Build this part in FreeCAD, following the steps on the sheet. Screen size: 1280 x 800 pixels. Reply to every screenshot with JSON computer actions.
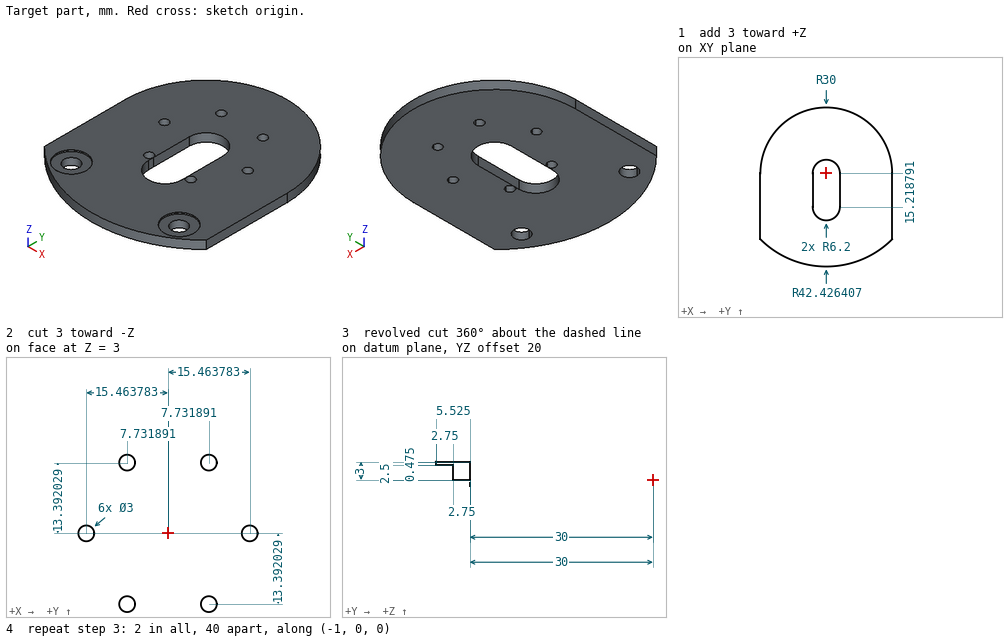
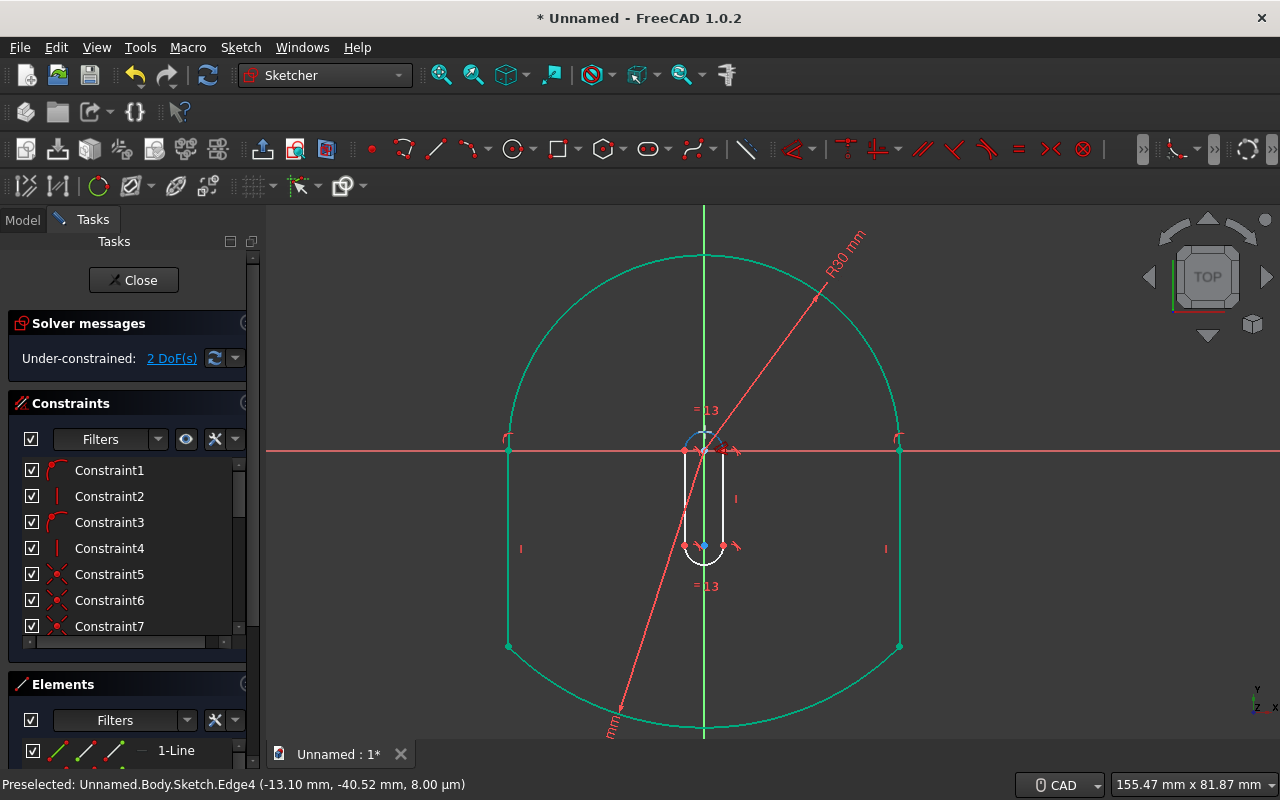
{"action": "left_click", "coordinate": [704, 432]}
{"action": "left_click", "coordinate": [728, 406]}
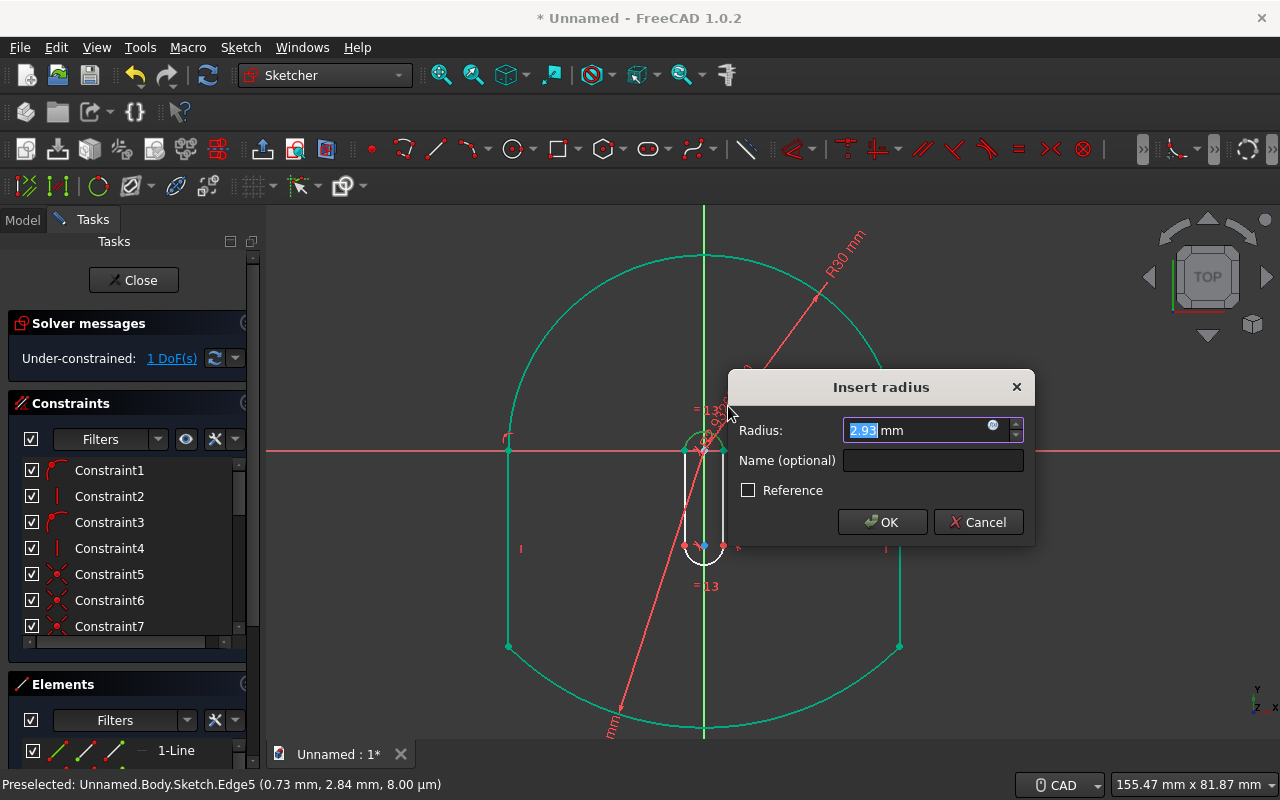
{"action": "type", "text": "6.2"}
{"action": "key", "text": "Return"}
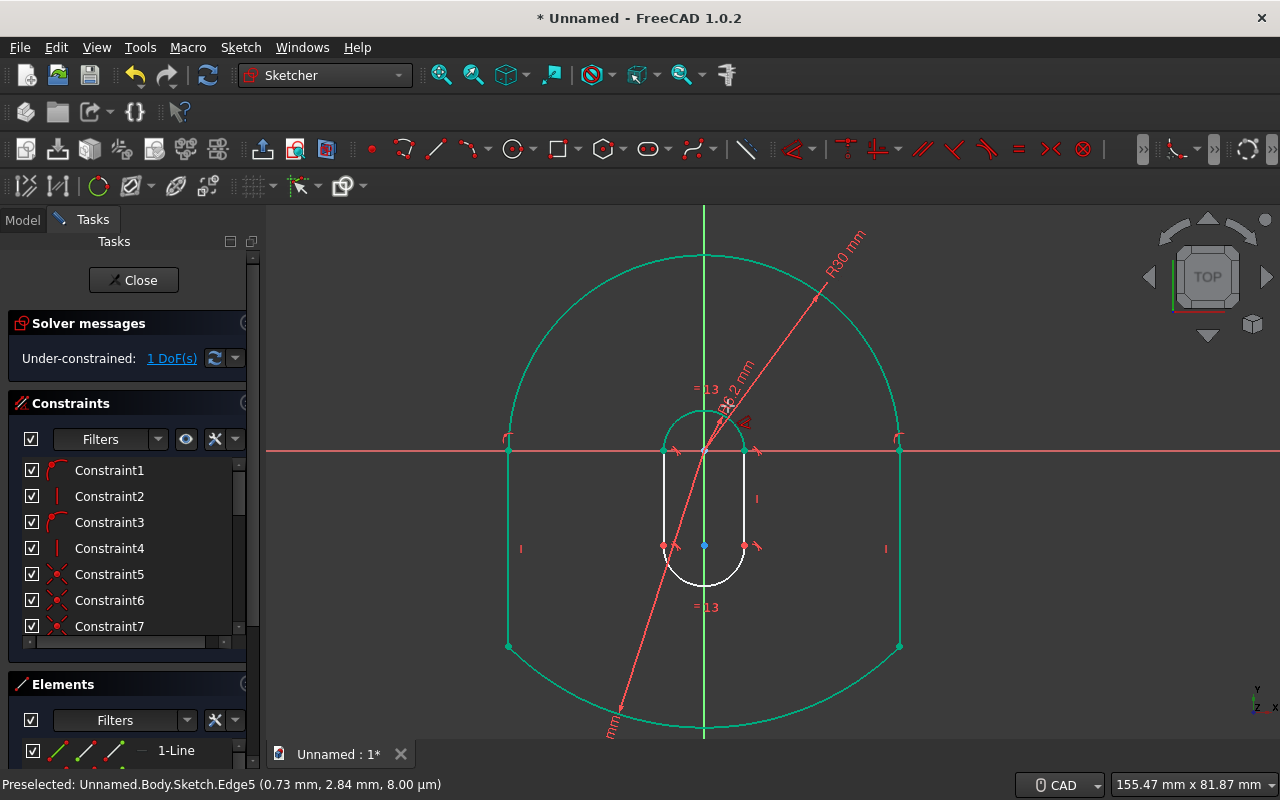
{"action": "left_click", "coordinate": [744, 479]}
{"action": "left_click", "coordinate": [778, 498]}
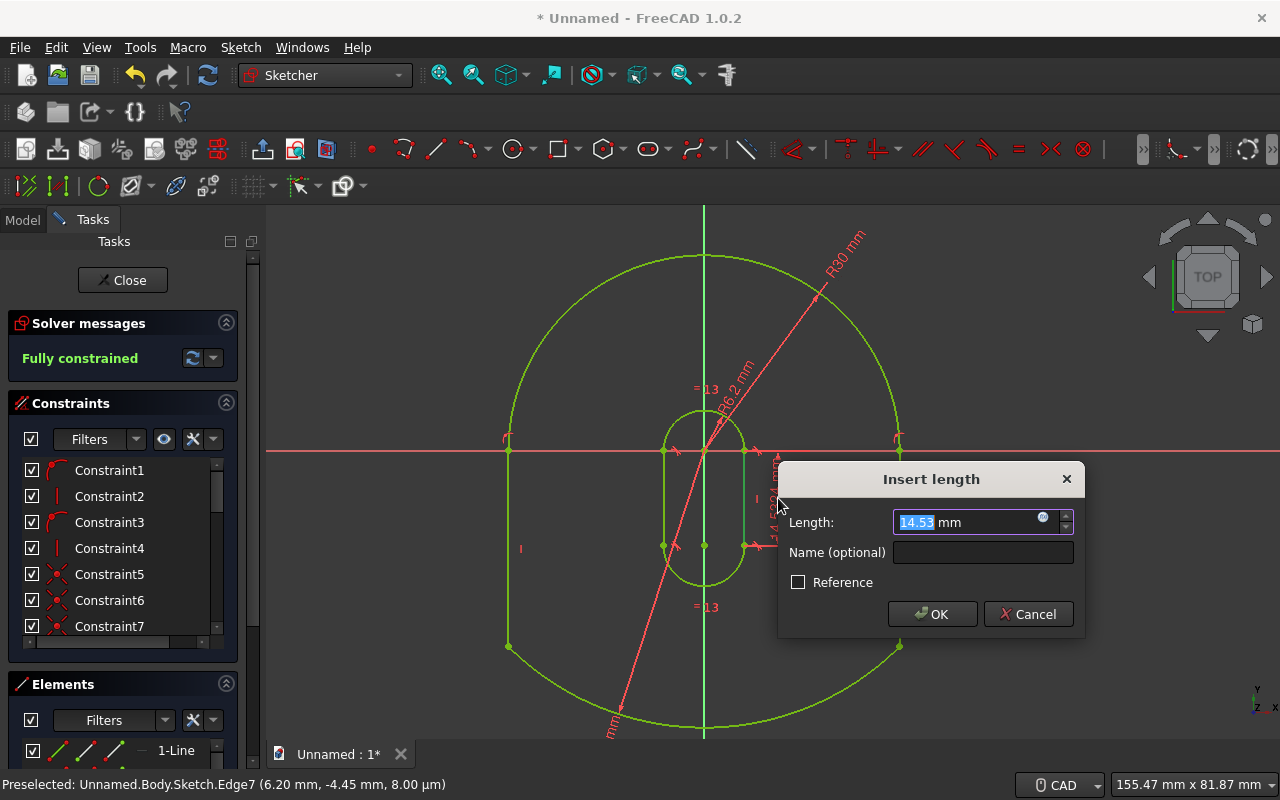
{"action": "type", "text": "15.218791"}
{"action": "key", "text": "Return"}
{"action": "key", "text": "Escape"}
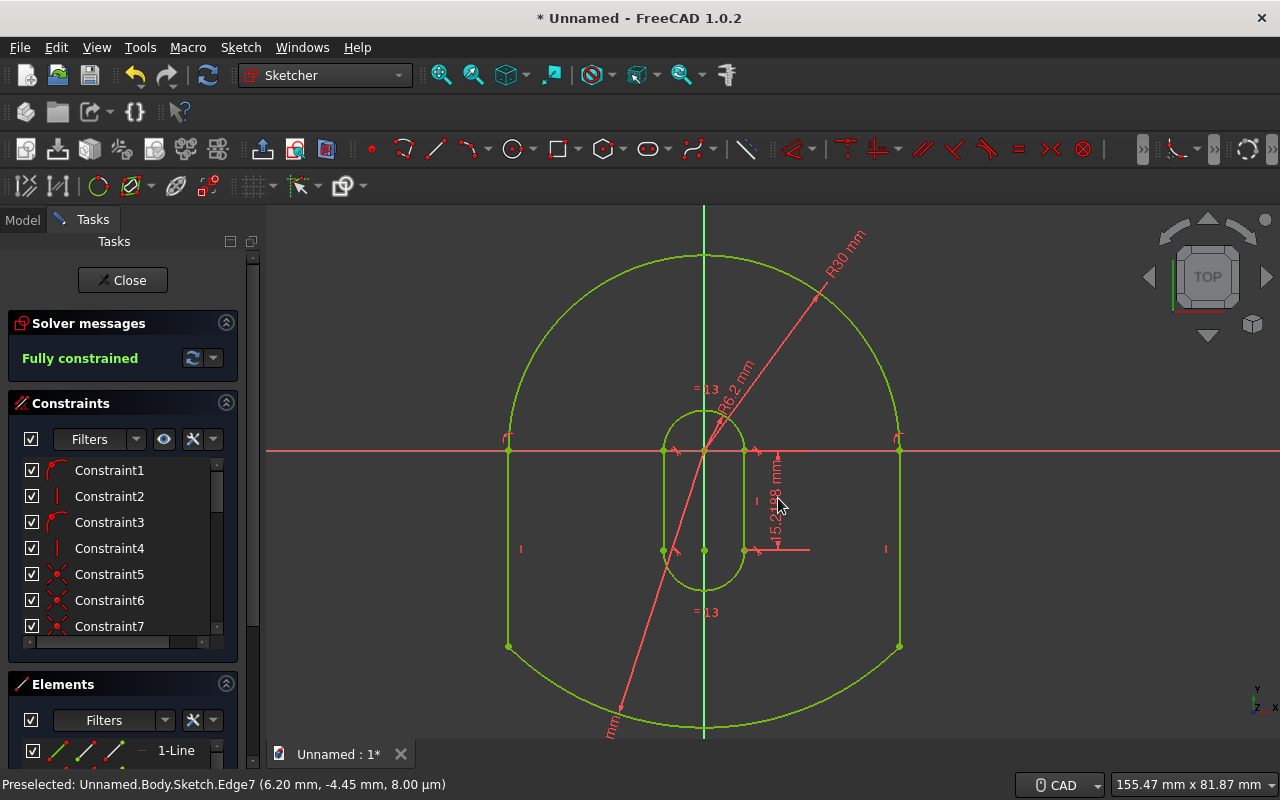
{"action": "left_click", "coordinate": [123, 280]}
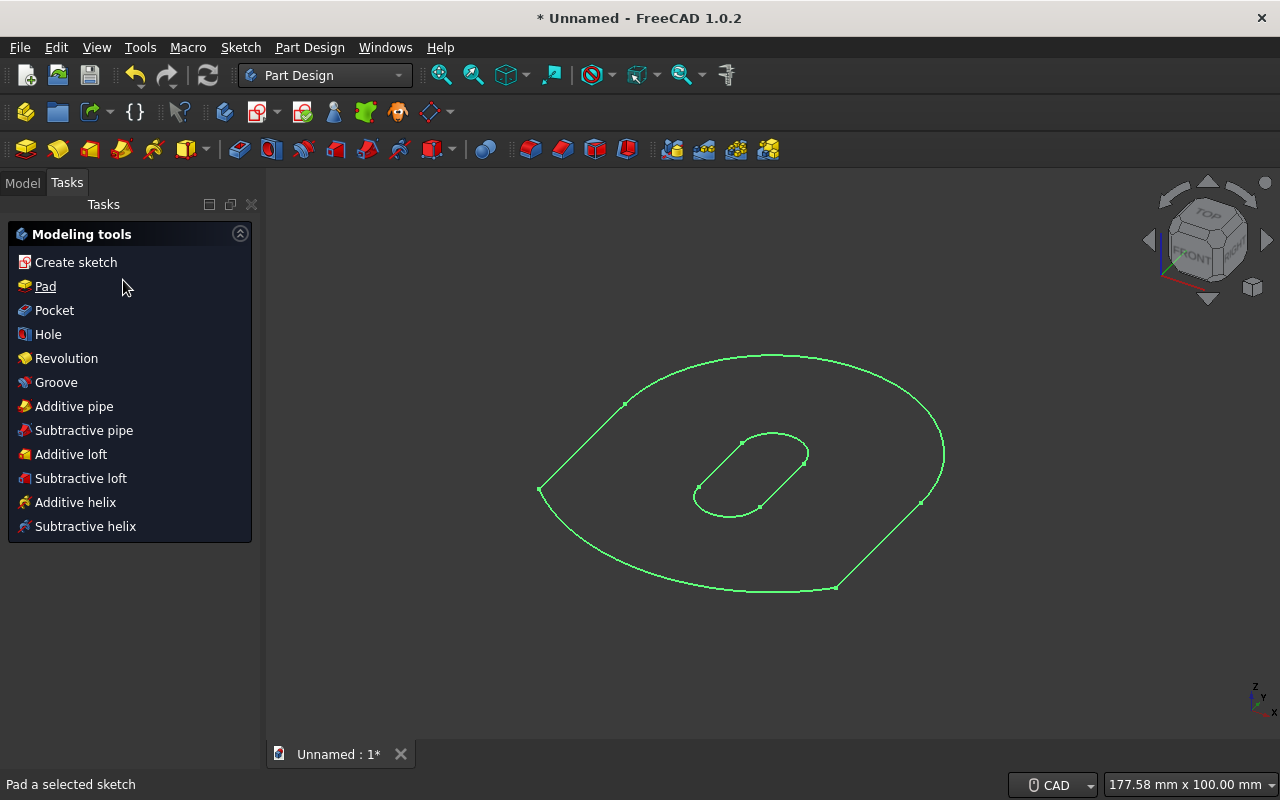
{"action": "left_click", "coordinate": [26, 150]}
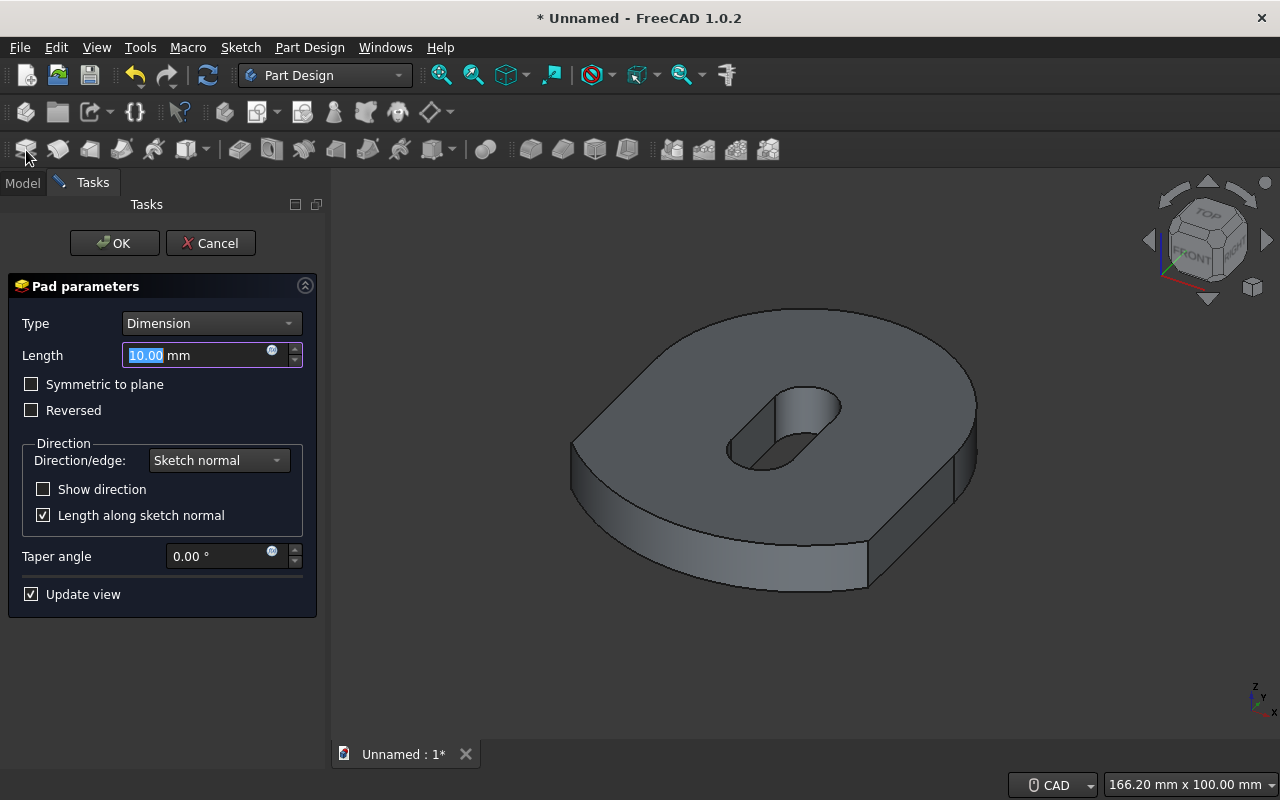
{"action": "type", "text": "3"}
{"action": "key", "text": "Tab"}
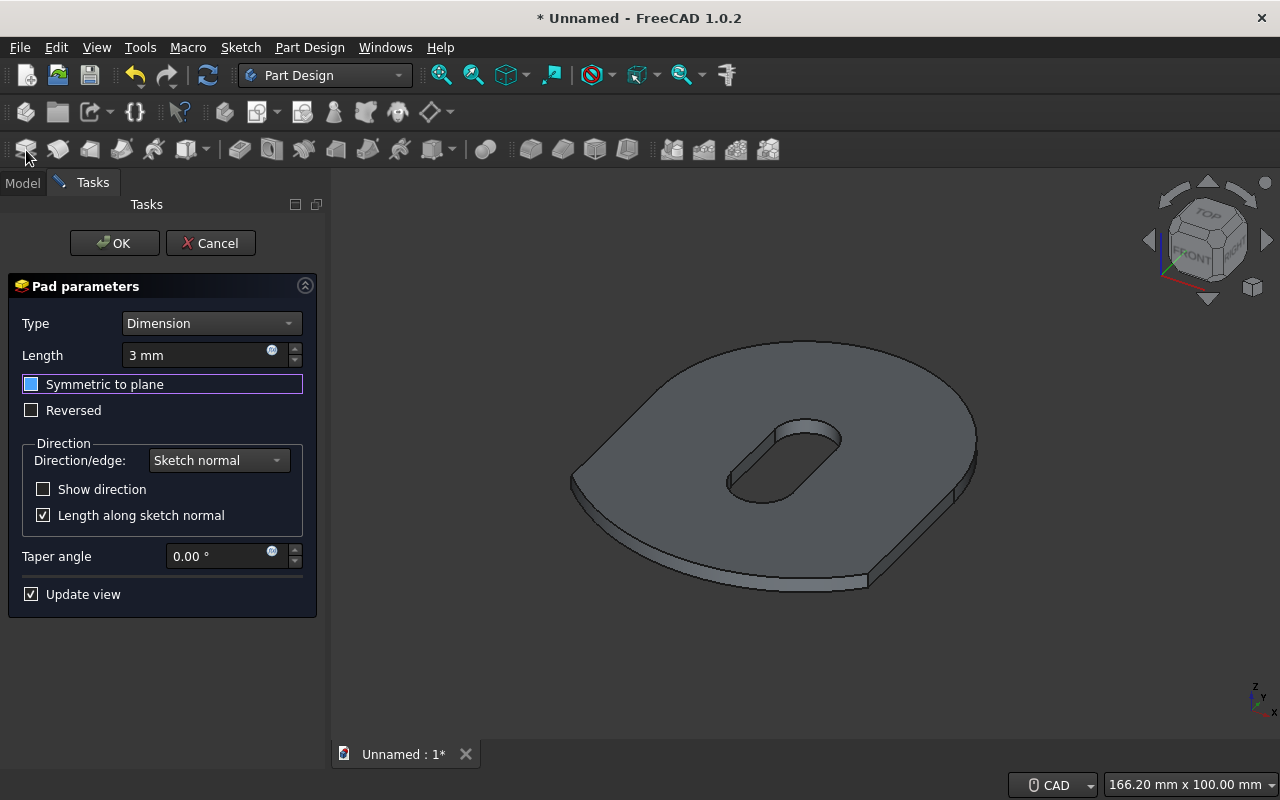
{"action": "left_click", "coordinate": [115, 243]}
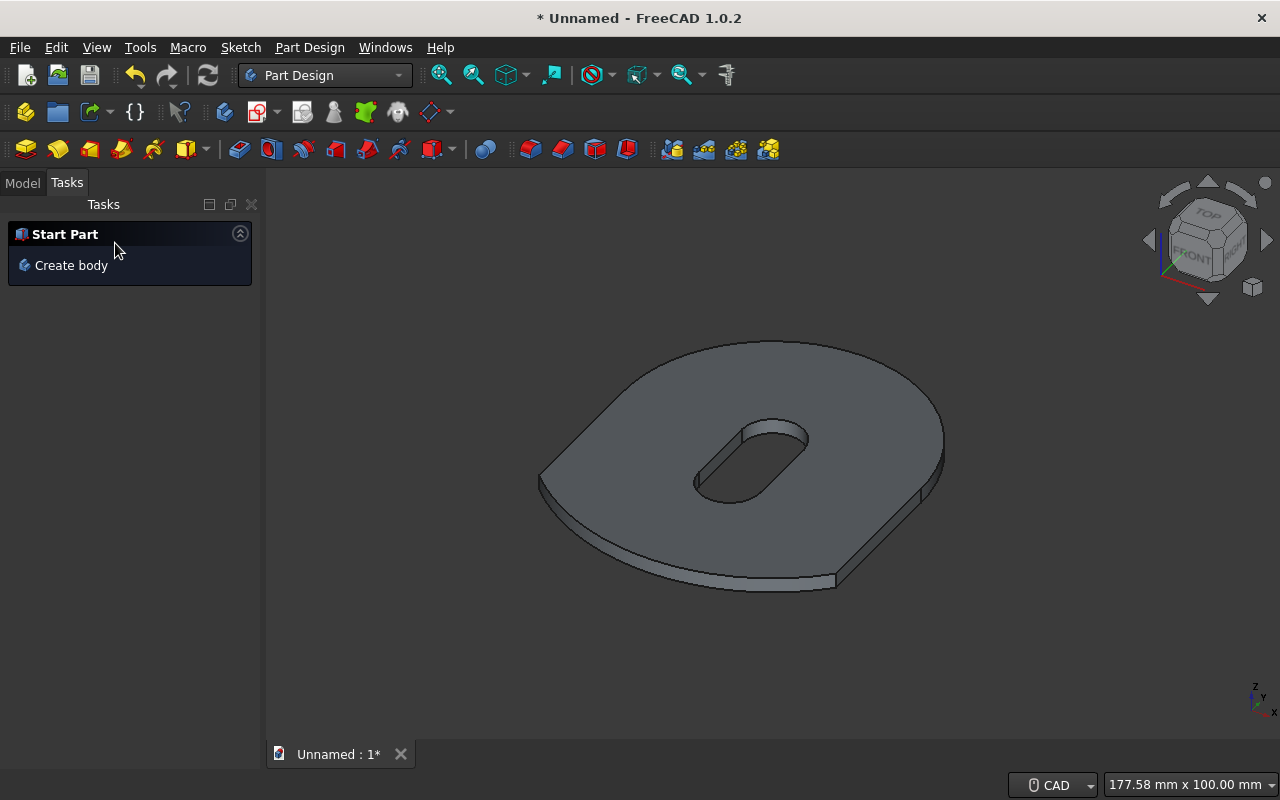
{"action": "left_click", "coordinate": [870, 455]}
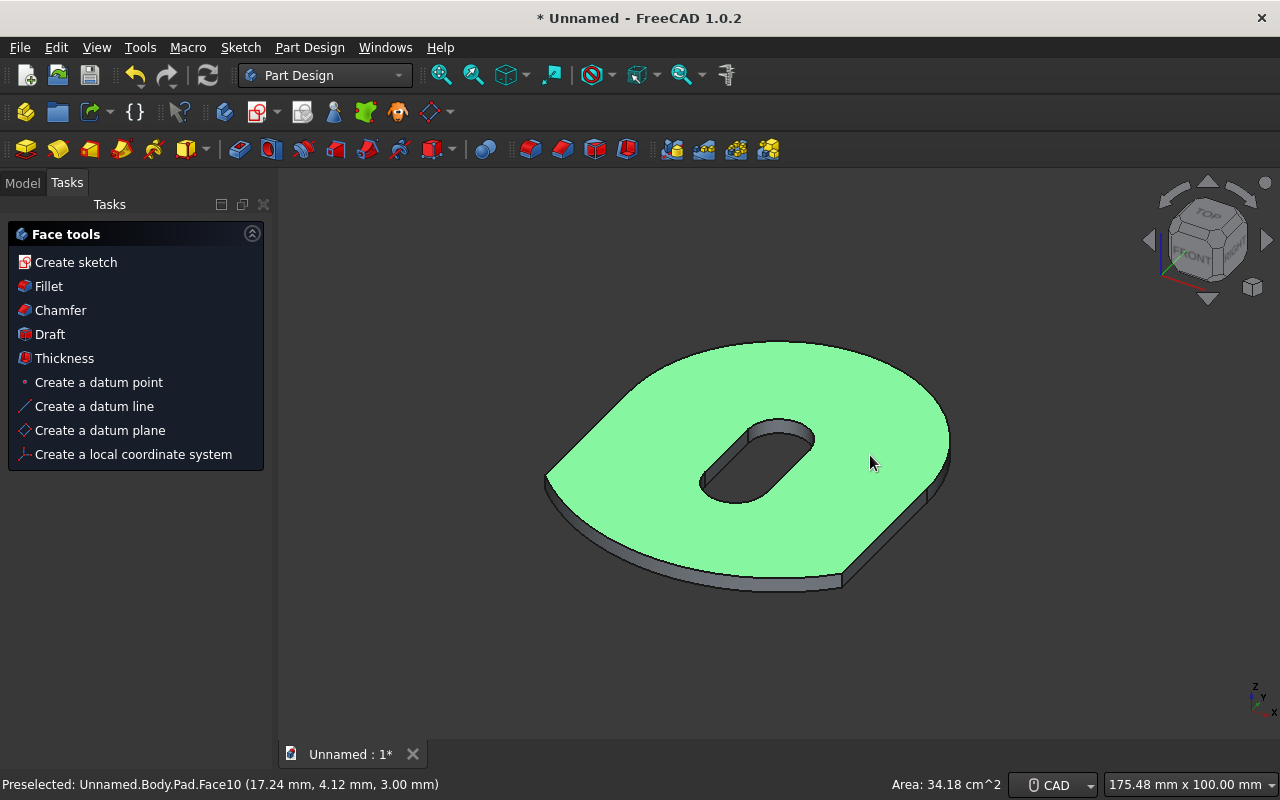
{"action": "left_click", "coordinate": [258, 112]}